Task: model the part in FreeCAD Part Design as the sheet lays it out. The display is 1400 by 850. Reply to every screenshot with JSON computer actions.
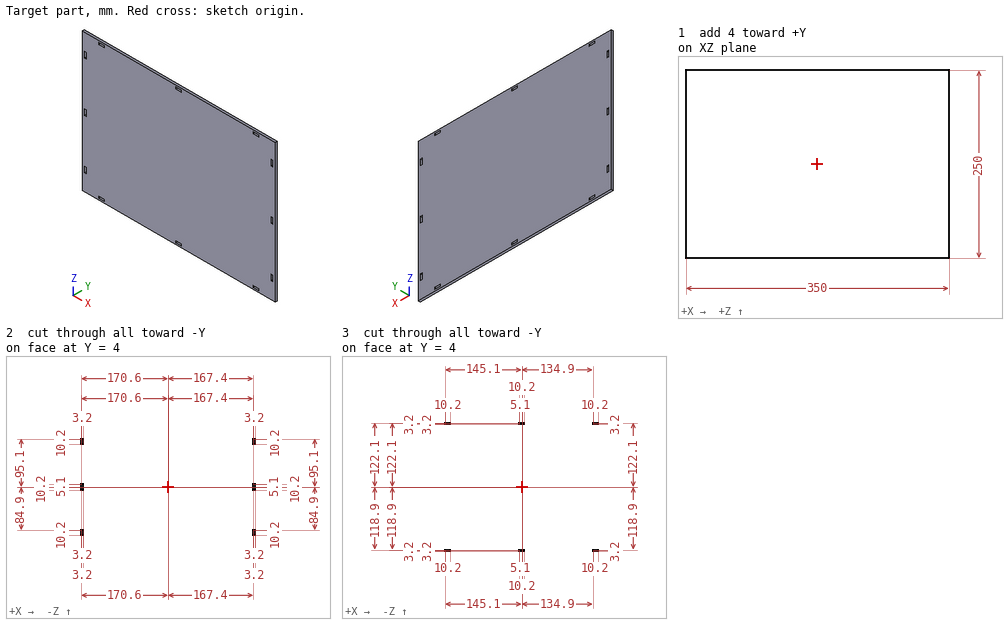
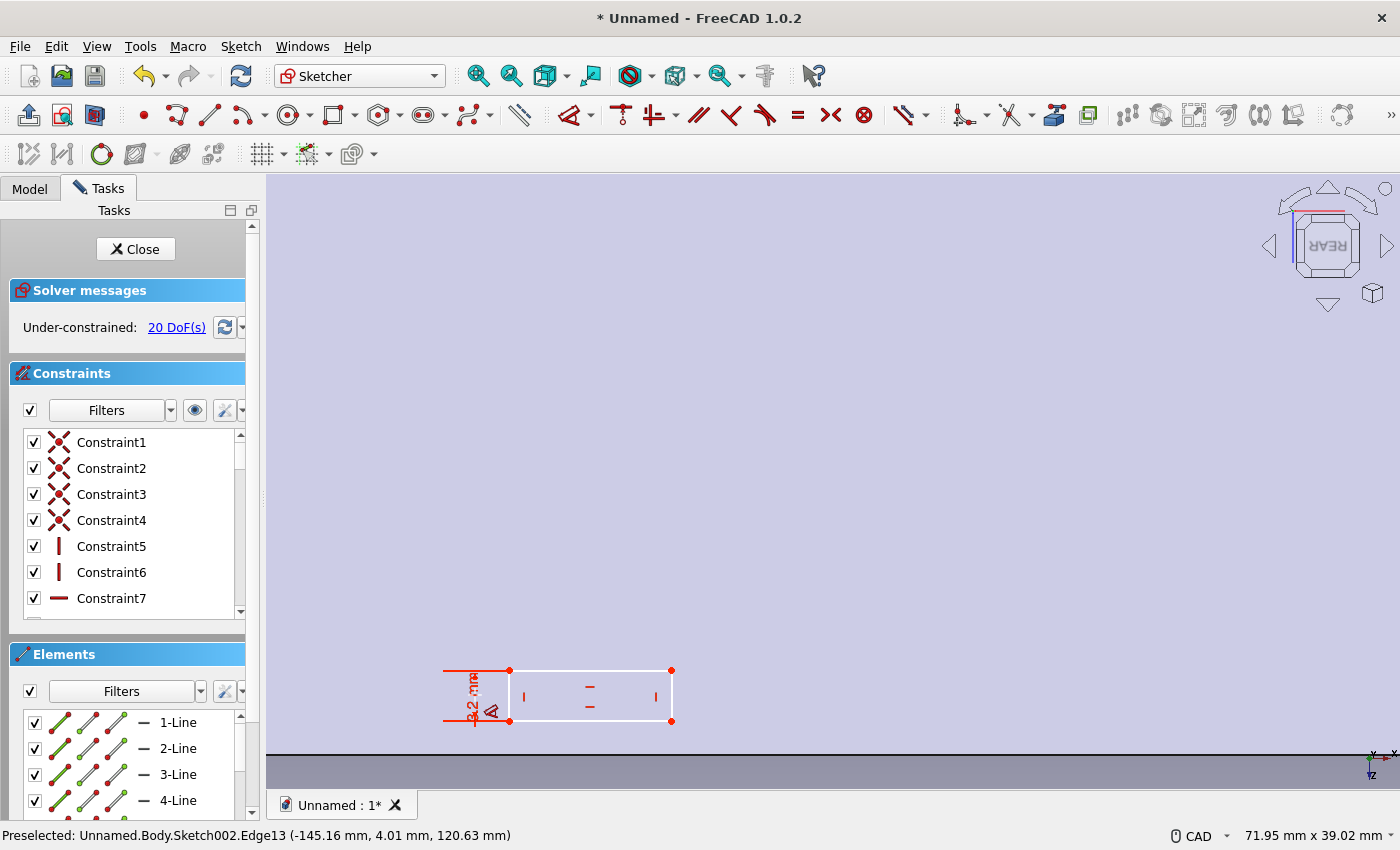
{"action": "scroll", "coordinate": [511, 693], "scroll_direction": "down", "scroll_amount": 11}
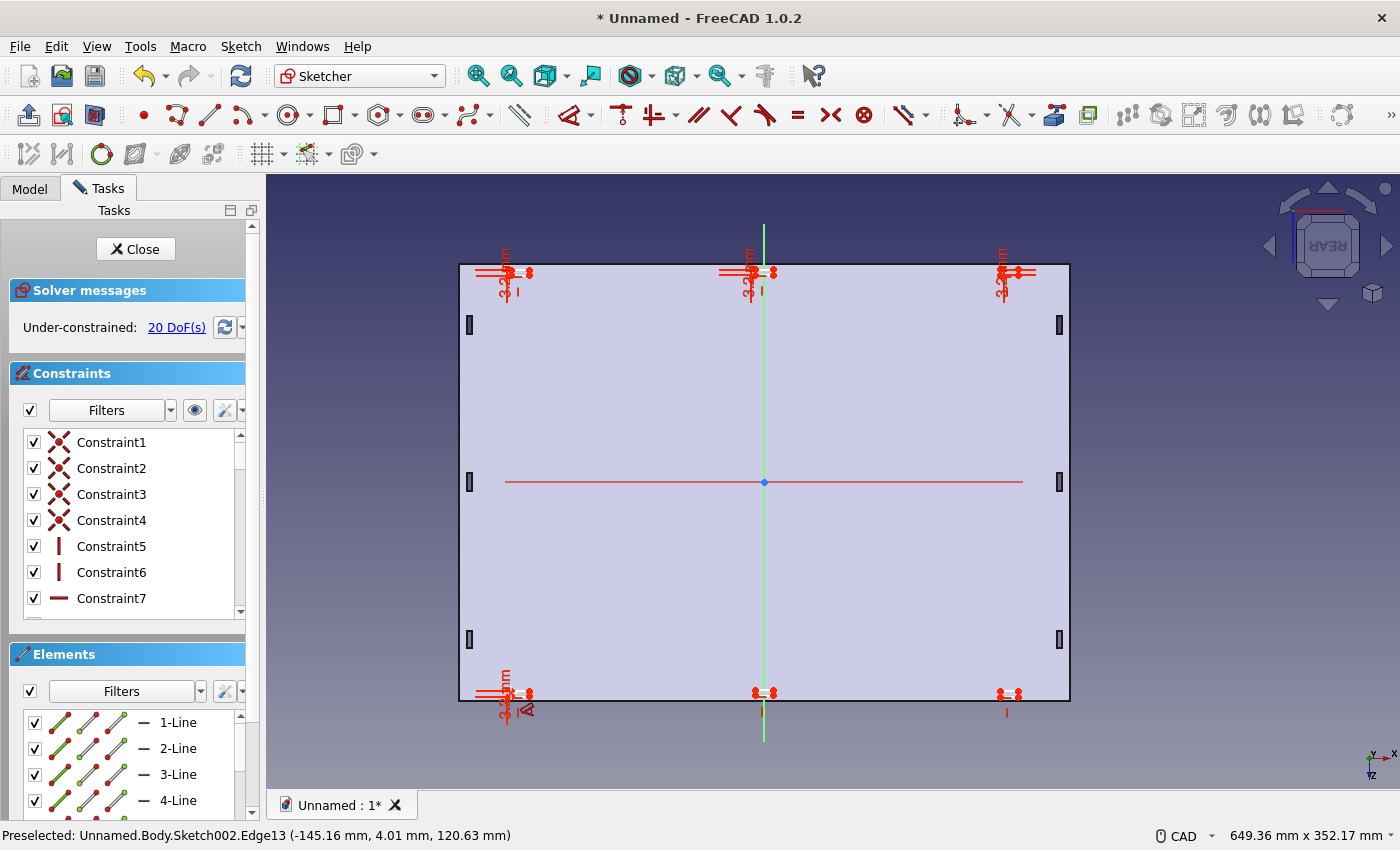
{"action": "scroll", "coordinate": [1000, 693], "scroll_direction": "up", "scroll_amount": 11}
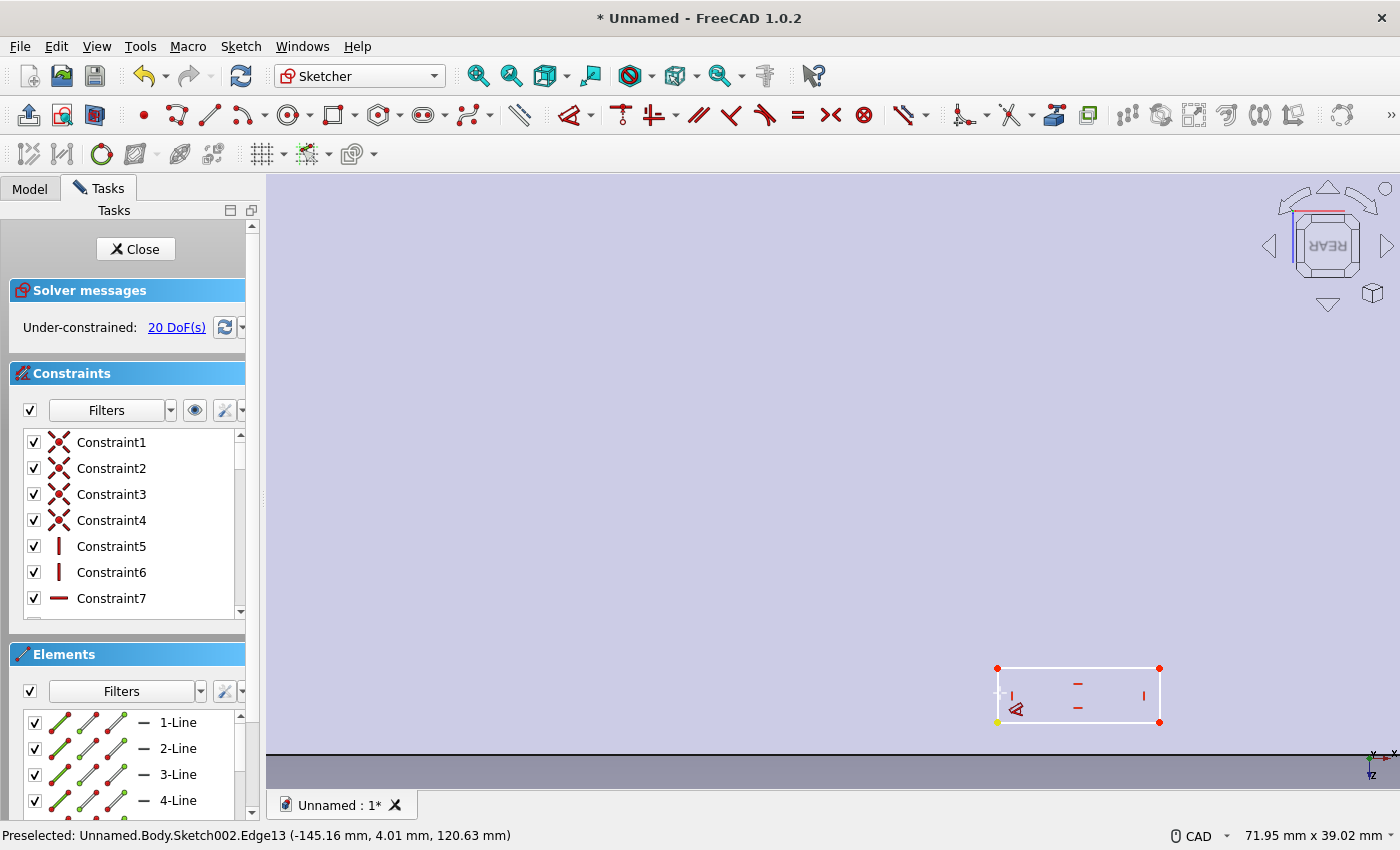
{"action": "left_click", "coordinate": [998, 685]}
{"action": "left_click", "coordinate": [1032, 695]}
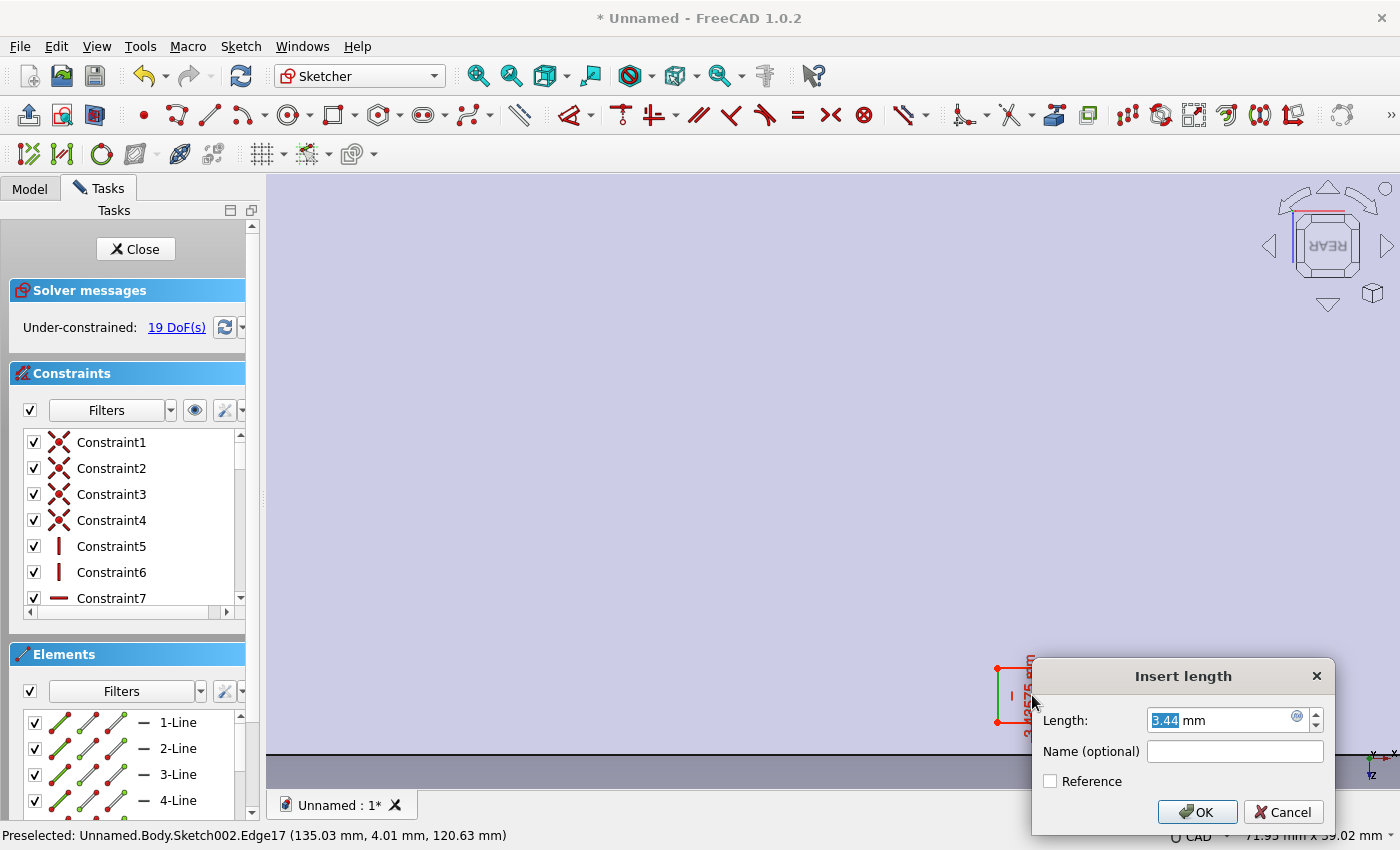
{"action": "type", "text": "3.2"}
{"action": "key", "text": "Return"}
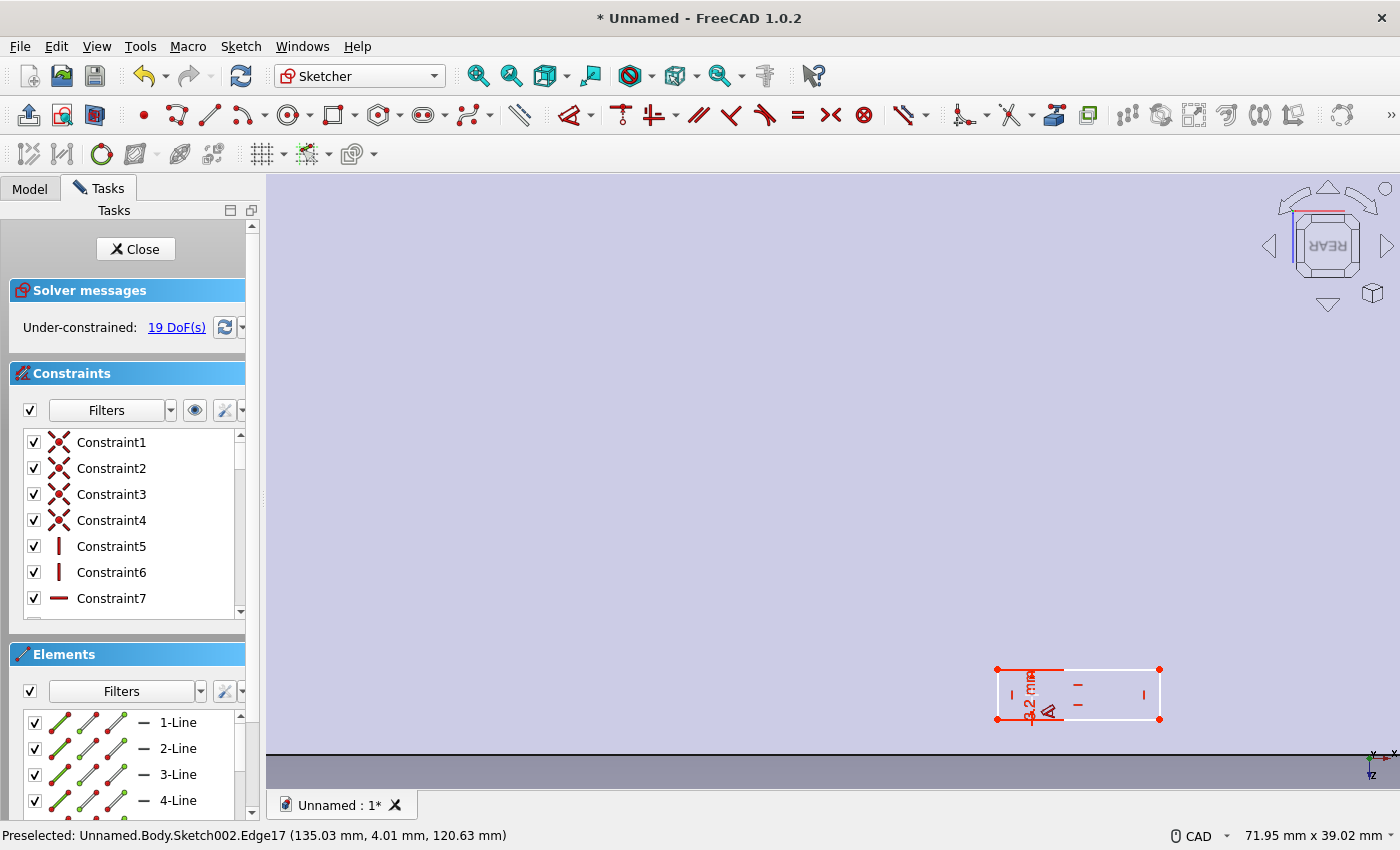
{"action": "scroll", "coordinate": [1001, 693], "scroll_direction": "down", "scroll_amount": 11}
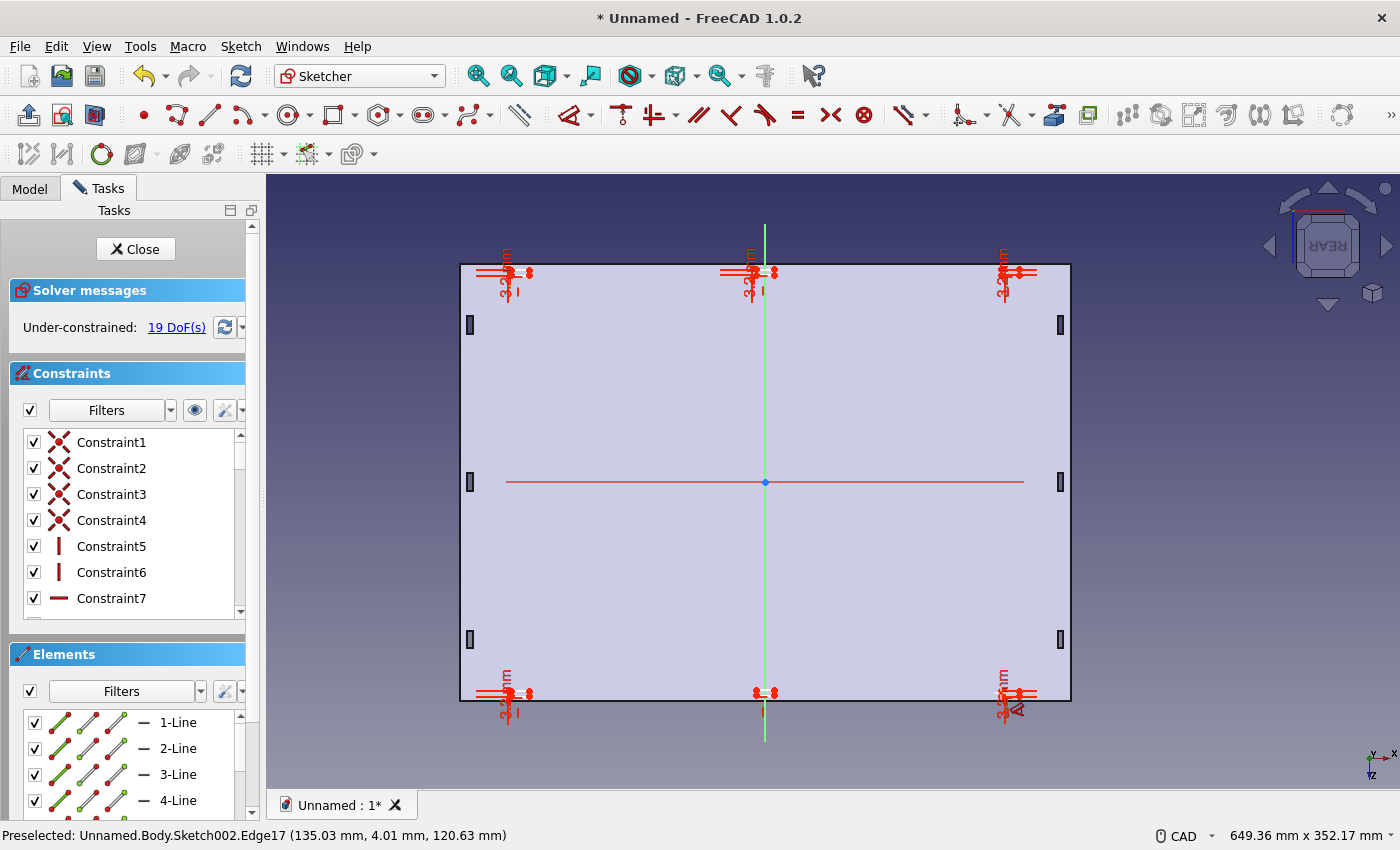
{"action": "scroll", "coordinate": [756, 692], "scroll_direction": "up", "scroll_amount": 11}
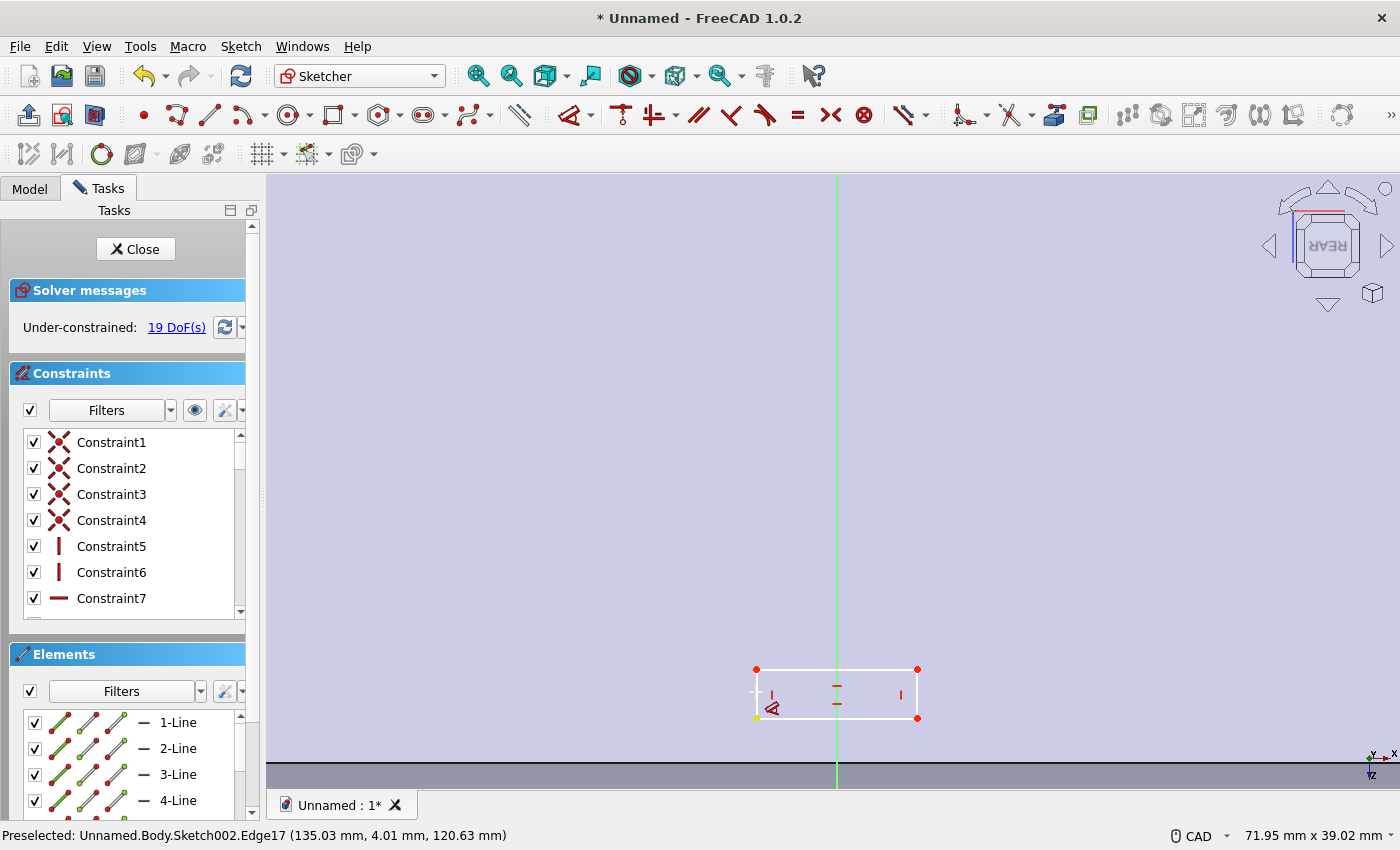
{"action": "left_click", "coordinate": [757, 685]}
{"action": "left_click", "coordinate": [723, 694]}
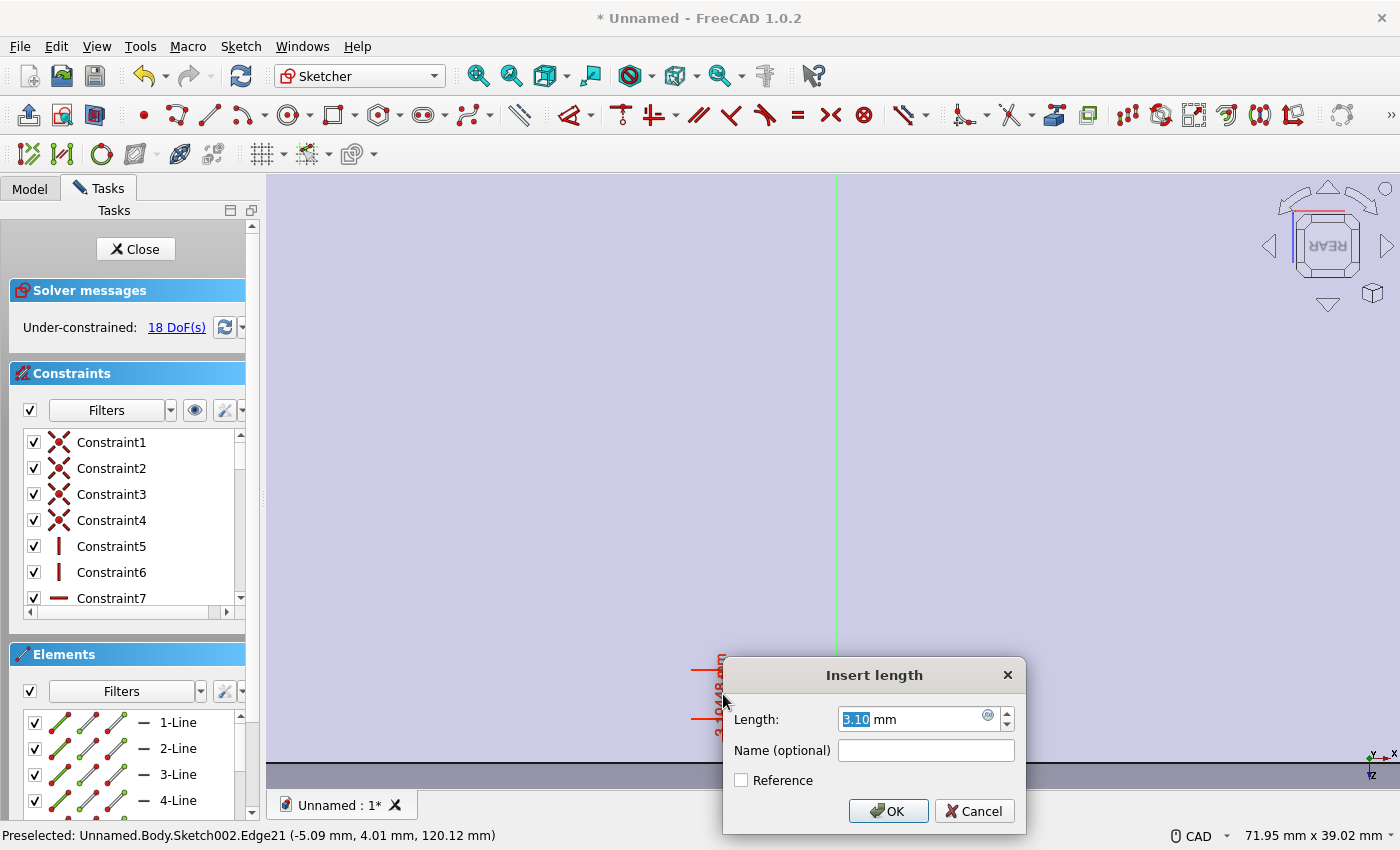
{"action": "type", "text": "3.2"}
{"action": "key", "text": "Return"}